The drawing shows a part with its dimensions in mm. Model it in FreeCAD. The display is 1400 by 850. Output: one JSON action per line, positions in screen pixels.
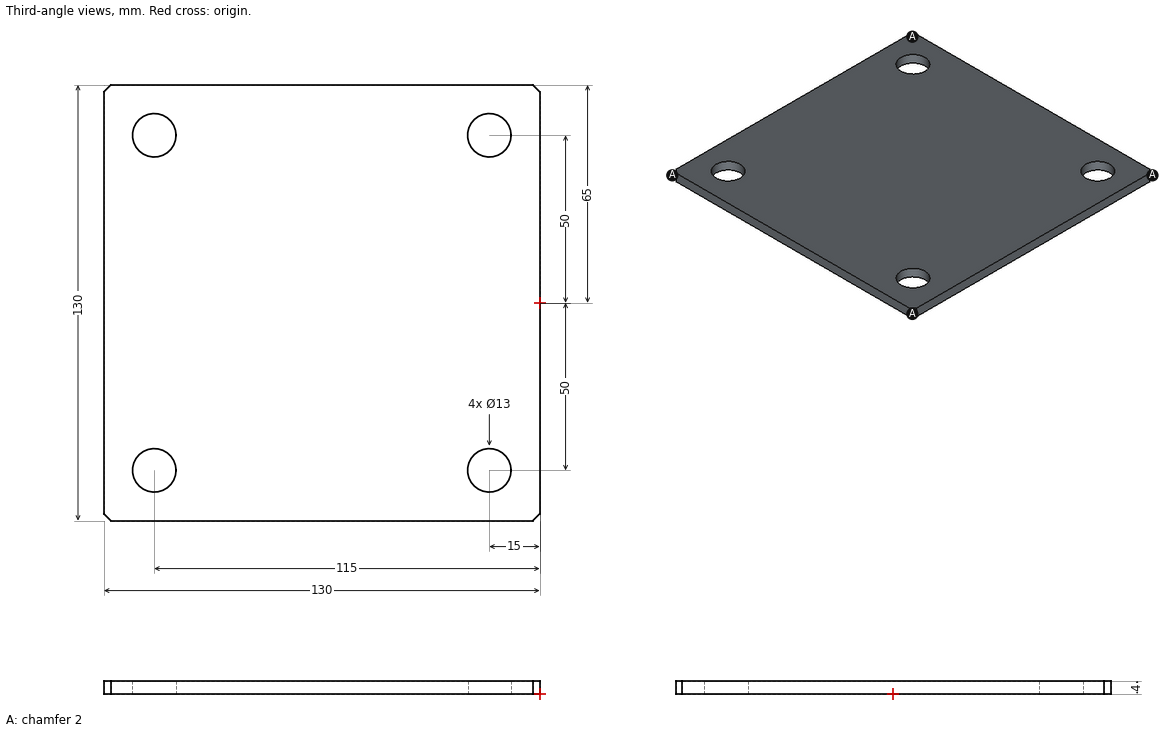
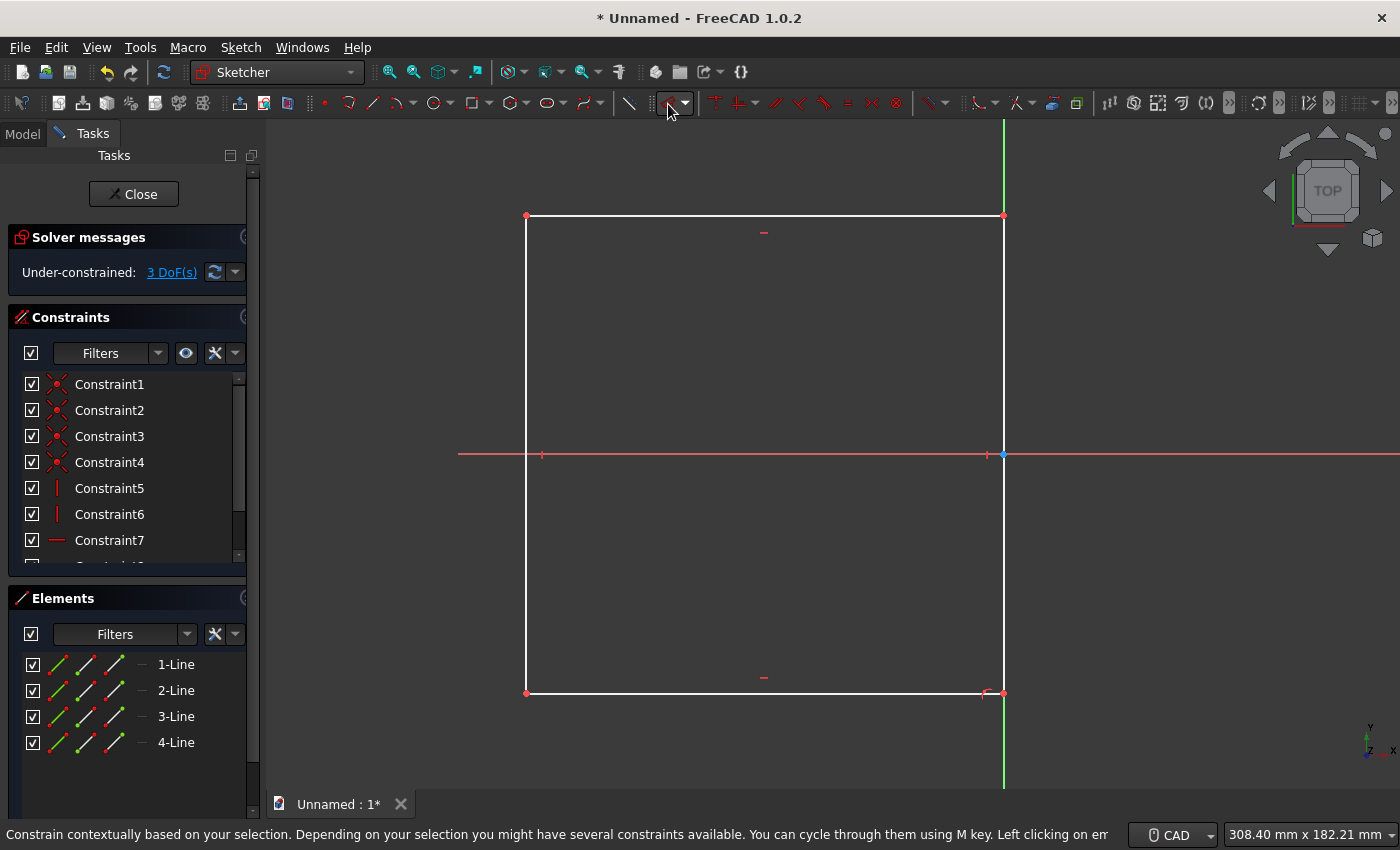
{"action": "left_click", "coordinate": [526, 359]}
{"action": "left_click", "coordinate": [492, 345]}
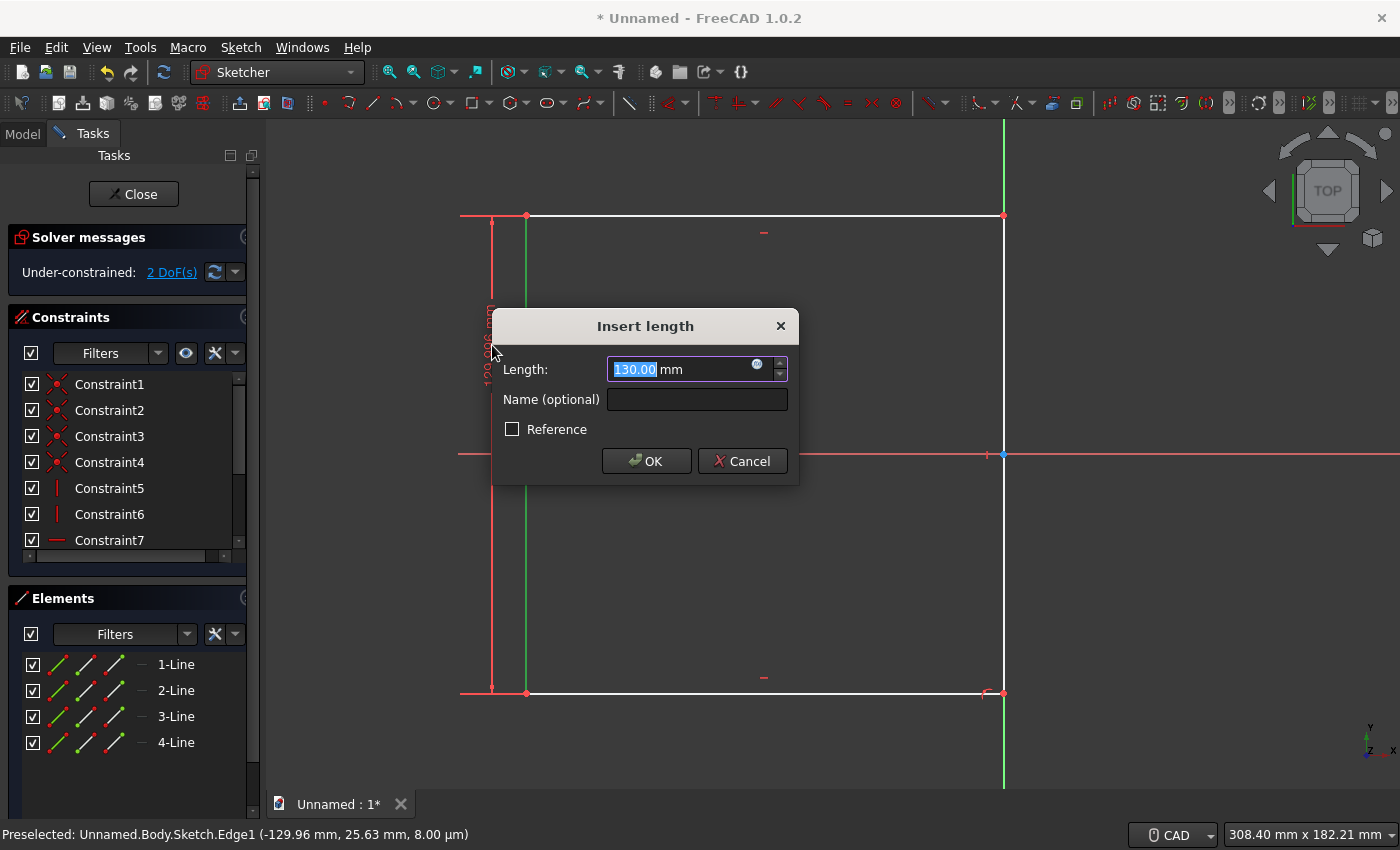
{"action": "type", "text": "130"}
{"action": "key", "text": "Return"}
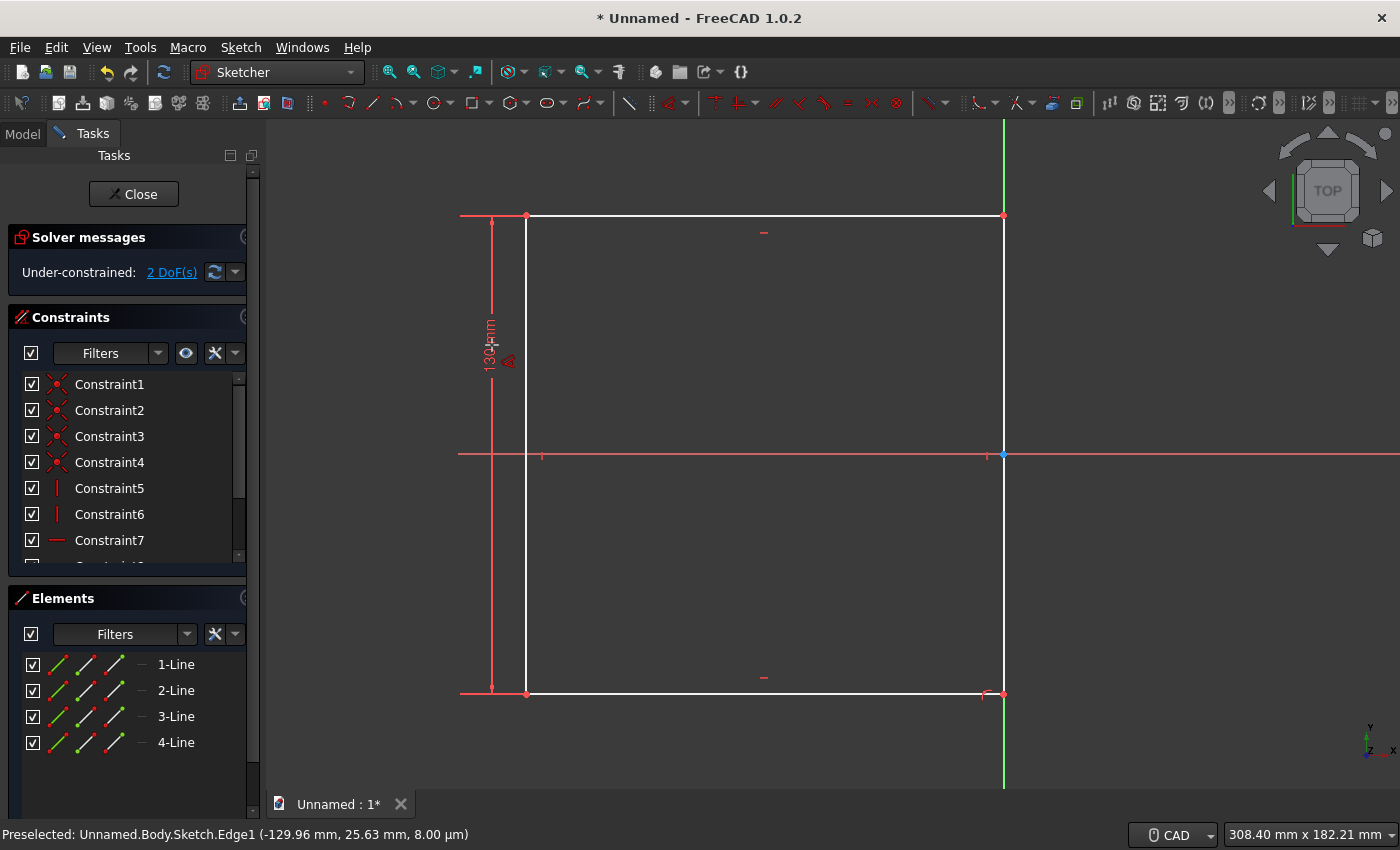
{"action": "left_click", "coordinate": [669, 694]}
{"action": "left_click", "coordinate": [765, 728]}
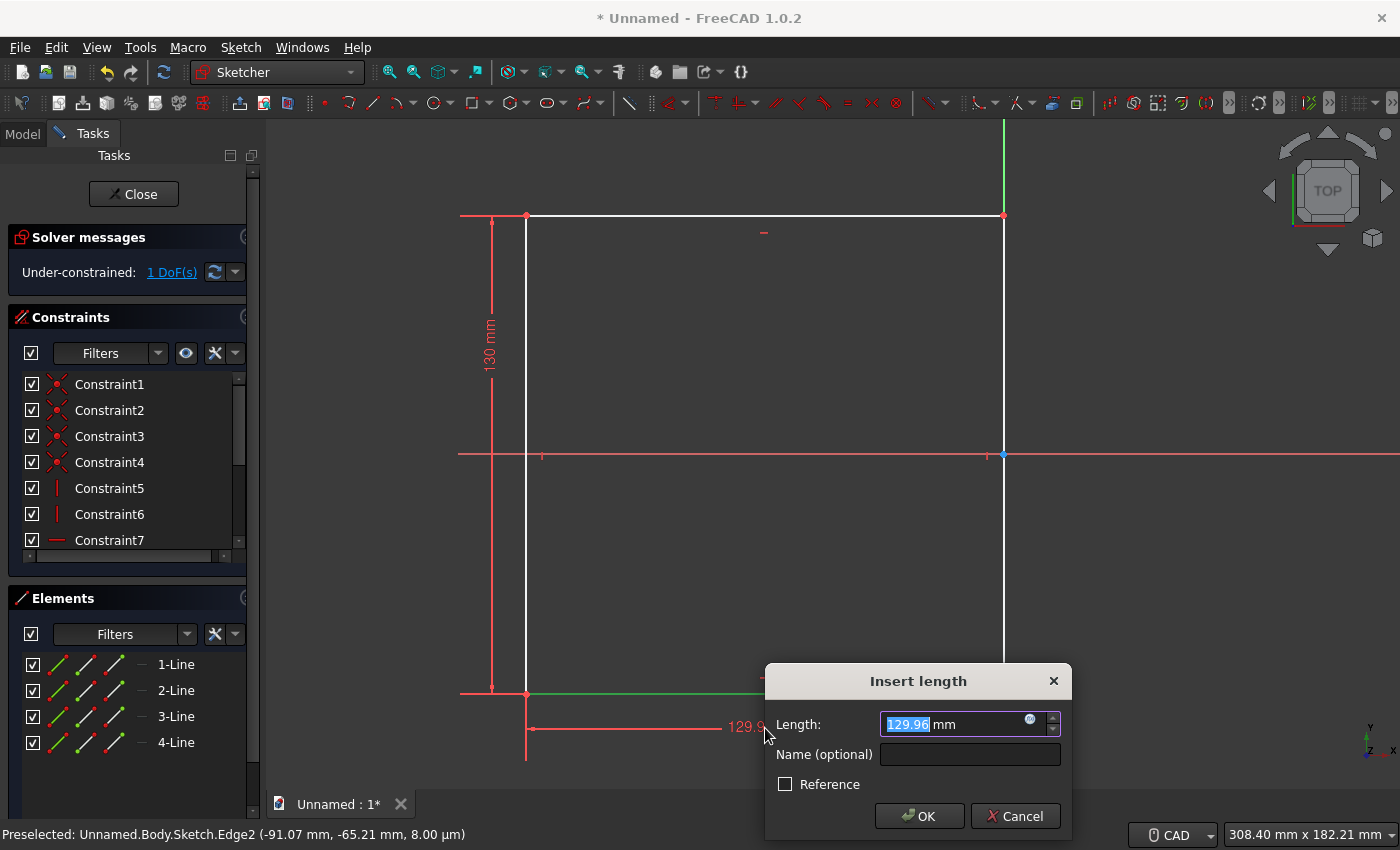
{"action": "type", "text": "130"}
{"action": "key", "text": "Return"}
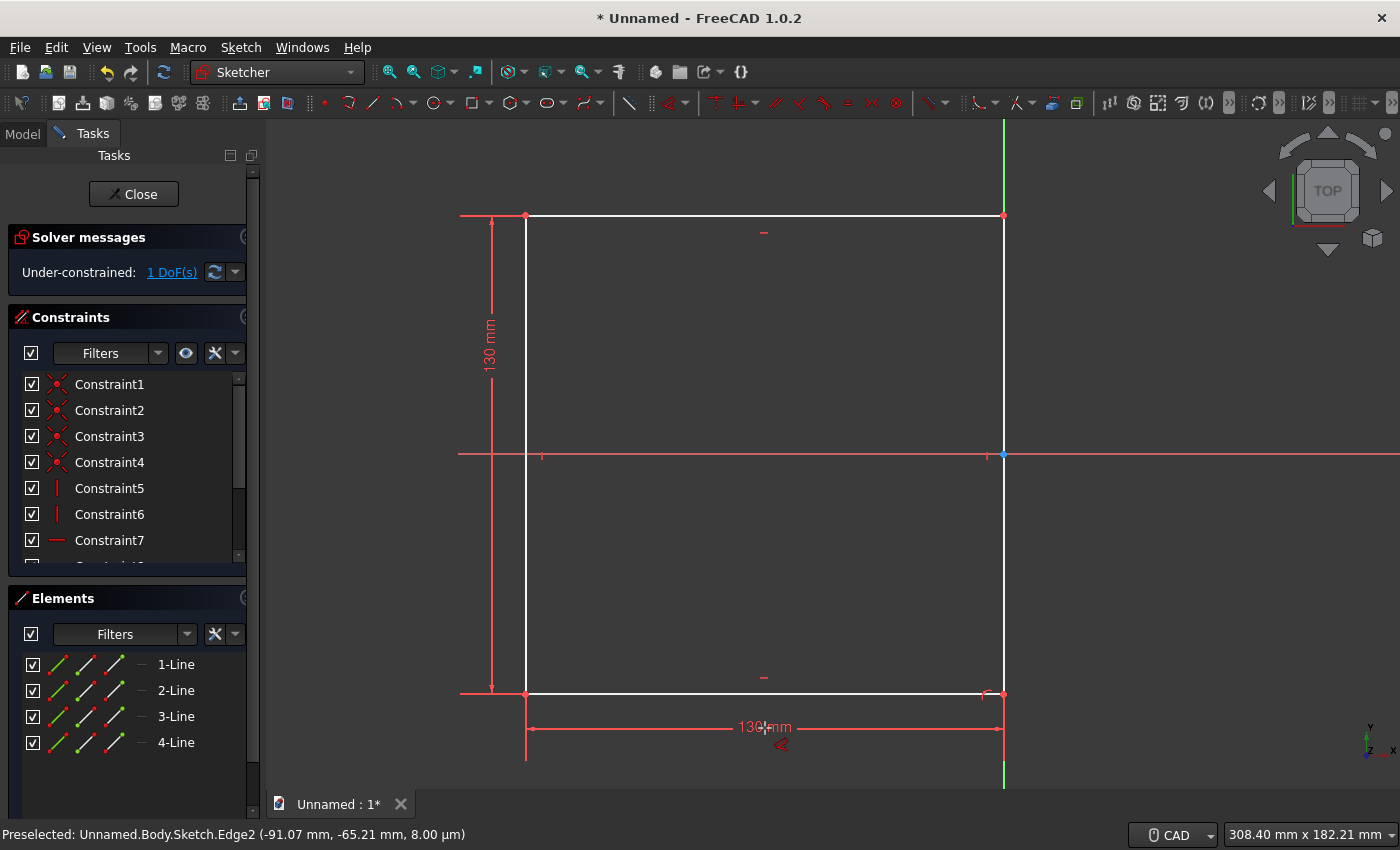
{"action": "left_click", "coordinate": [526, 216]}
{"action": "left_click", "coordinate": [1038, 335]}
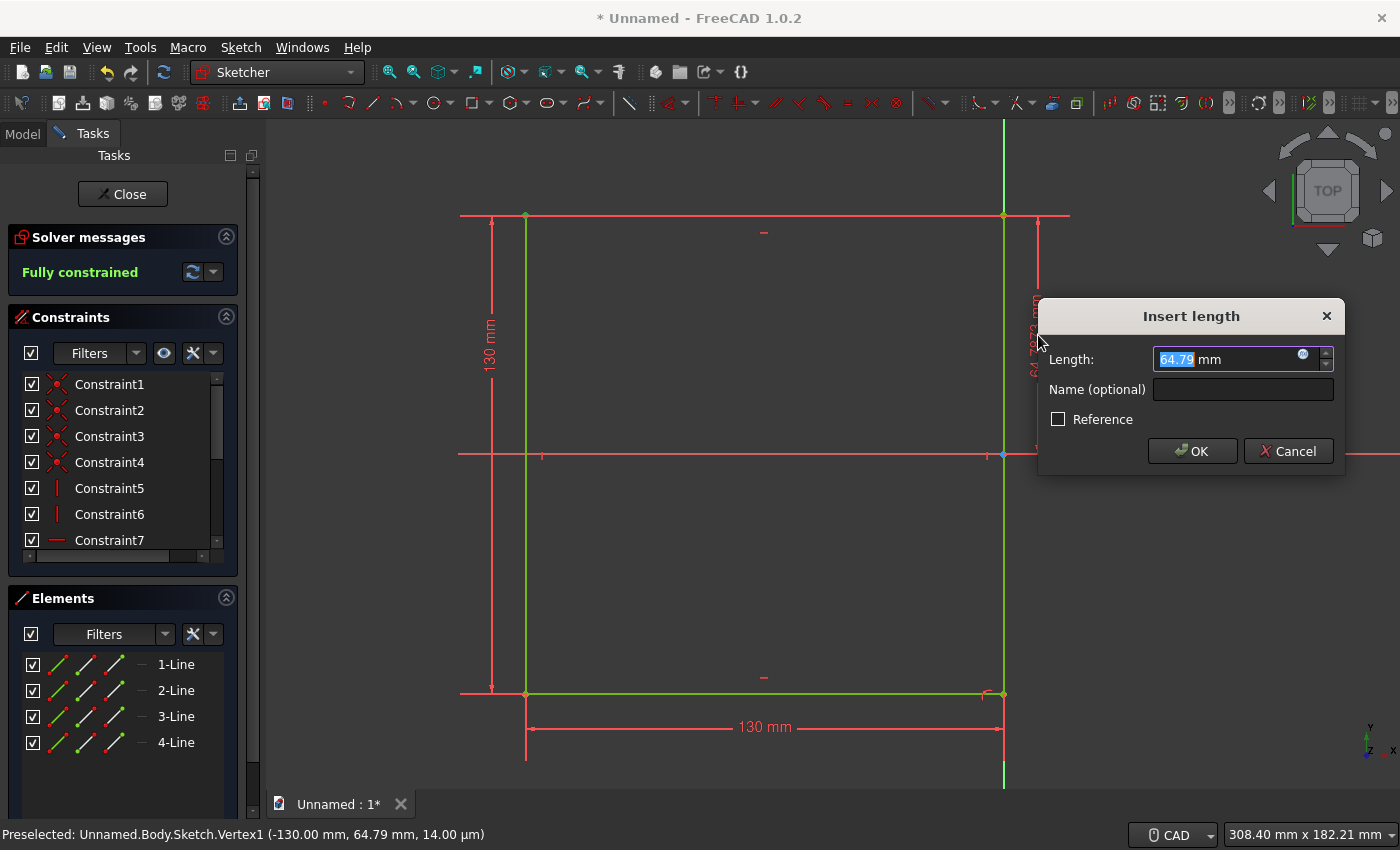
{"action": "type", "text": "65"}
{"action": "key", "text": "Return"}
{"action": "key", "text": "Escape"}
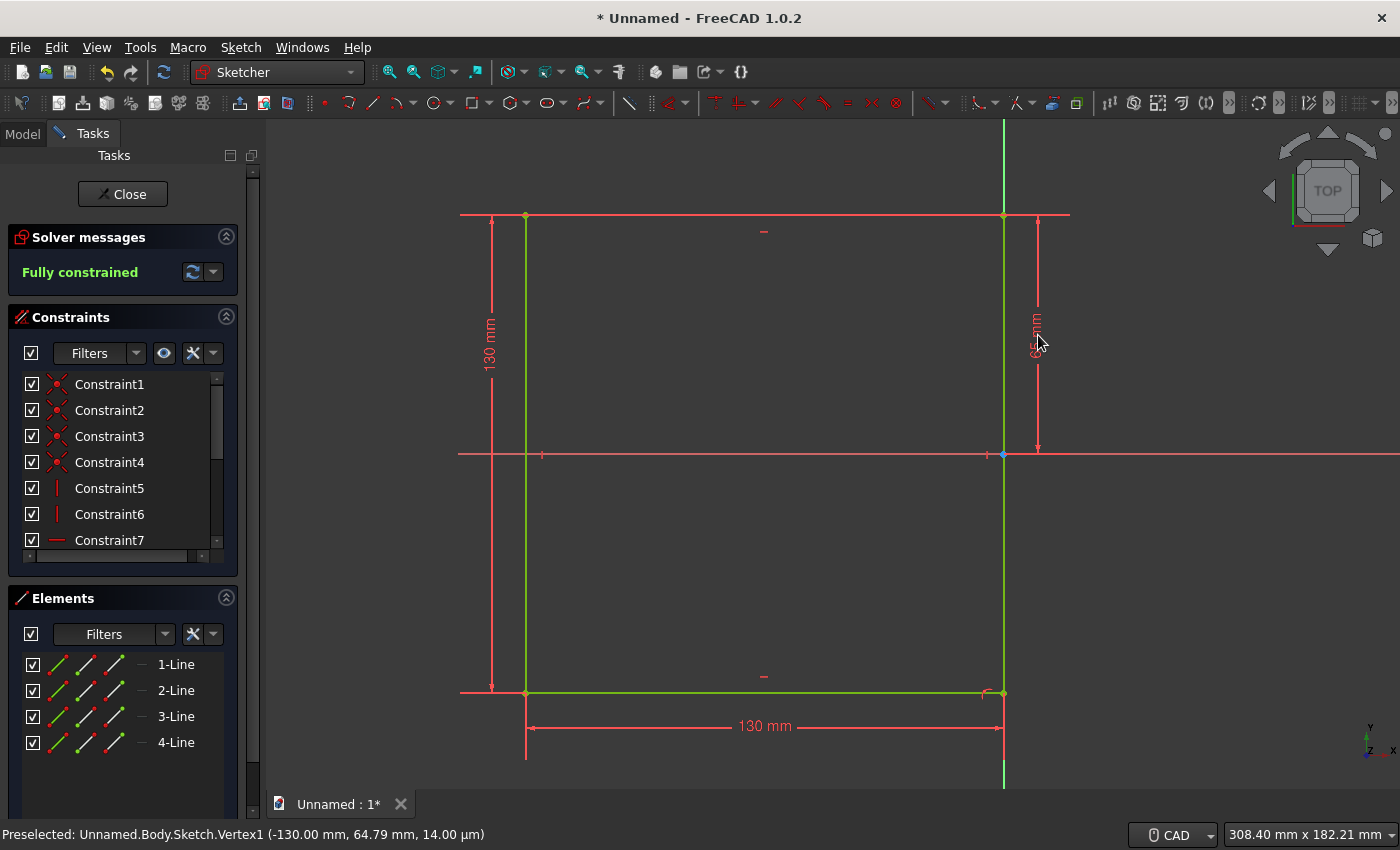
{"action": "left_click", "coordinate": [123, 194]}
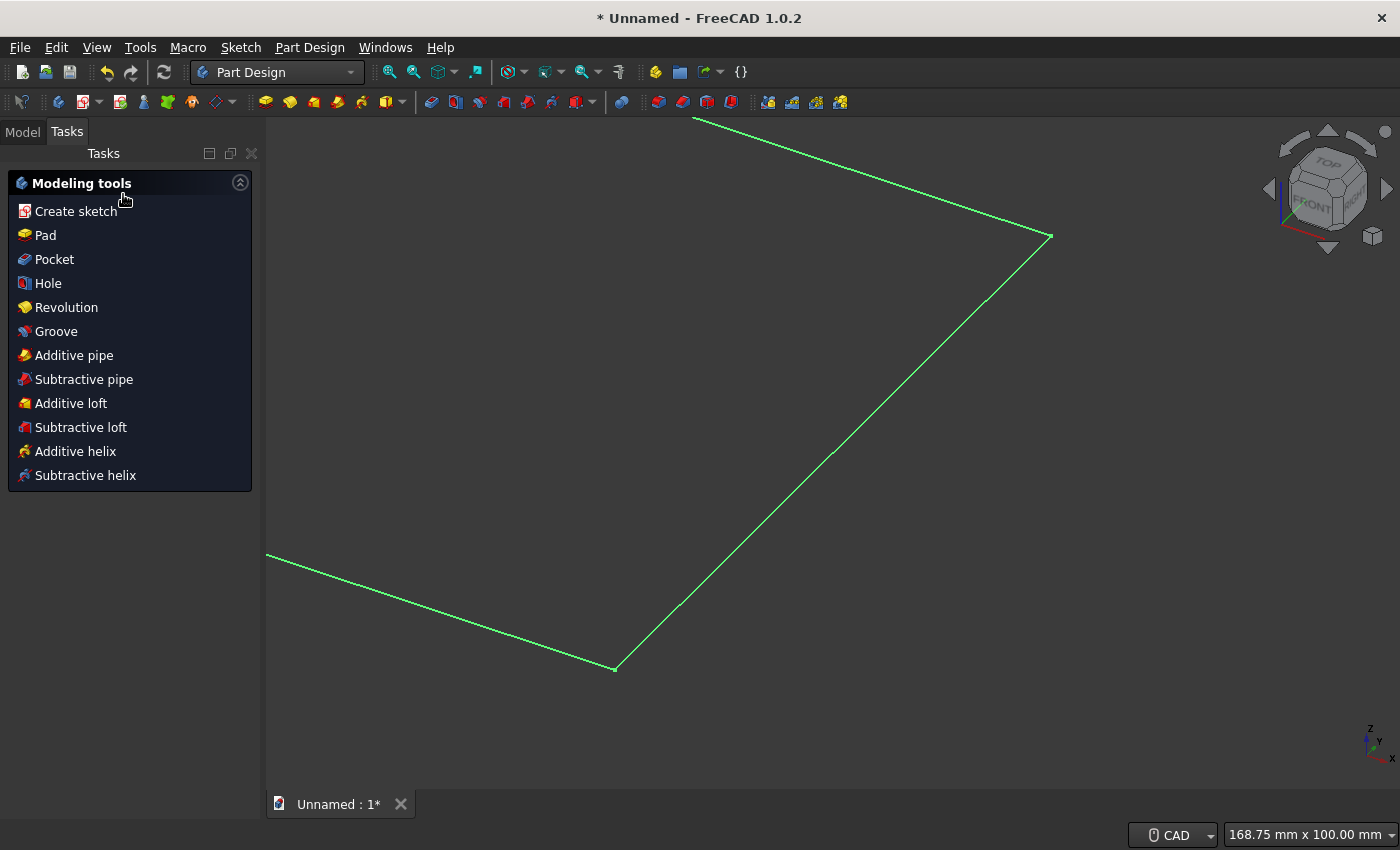
{"action": "left_click", "coordinate": [266, 102]}